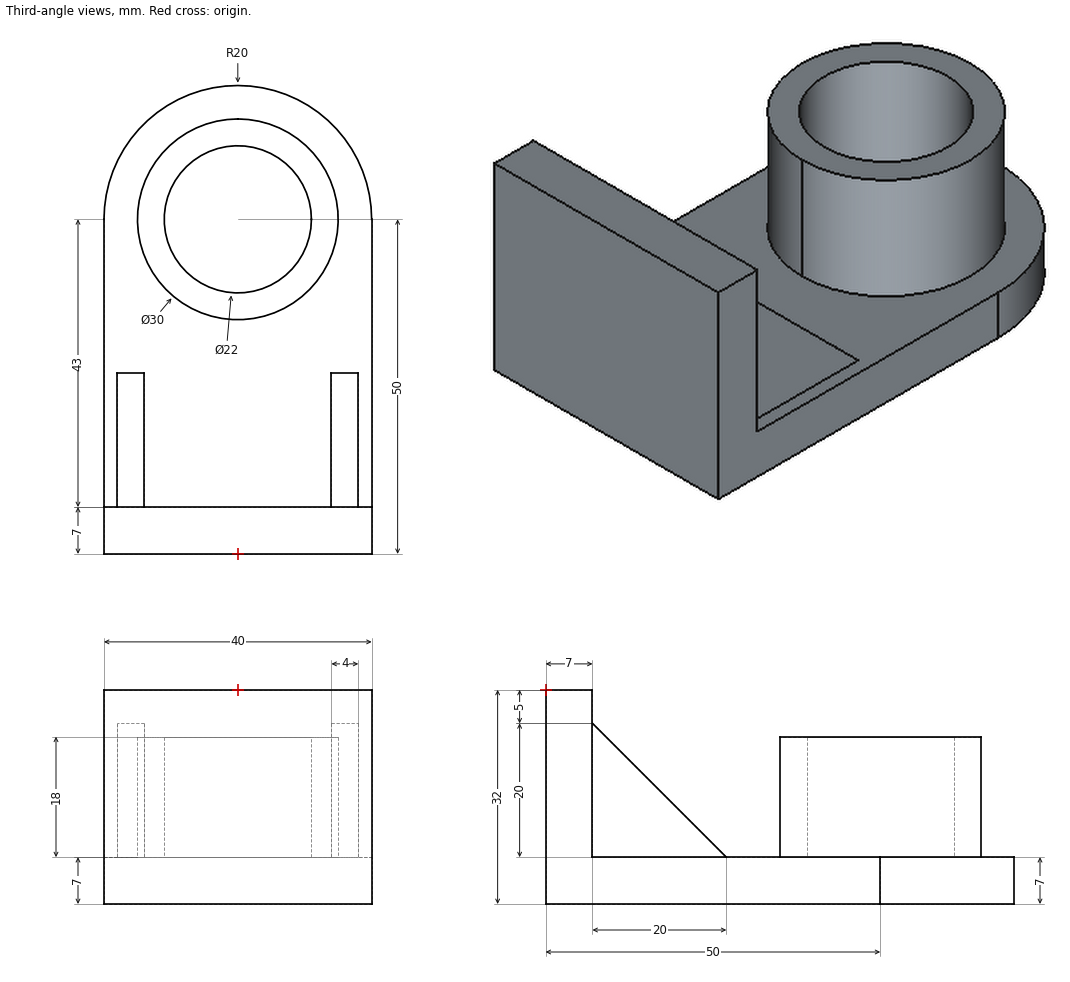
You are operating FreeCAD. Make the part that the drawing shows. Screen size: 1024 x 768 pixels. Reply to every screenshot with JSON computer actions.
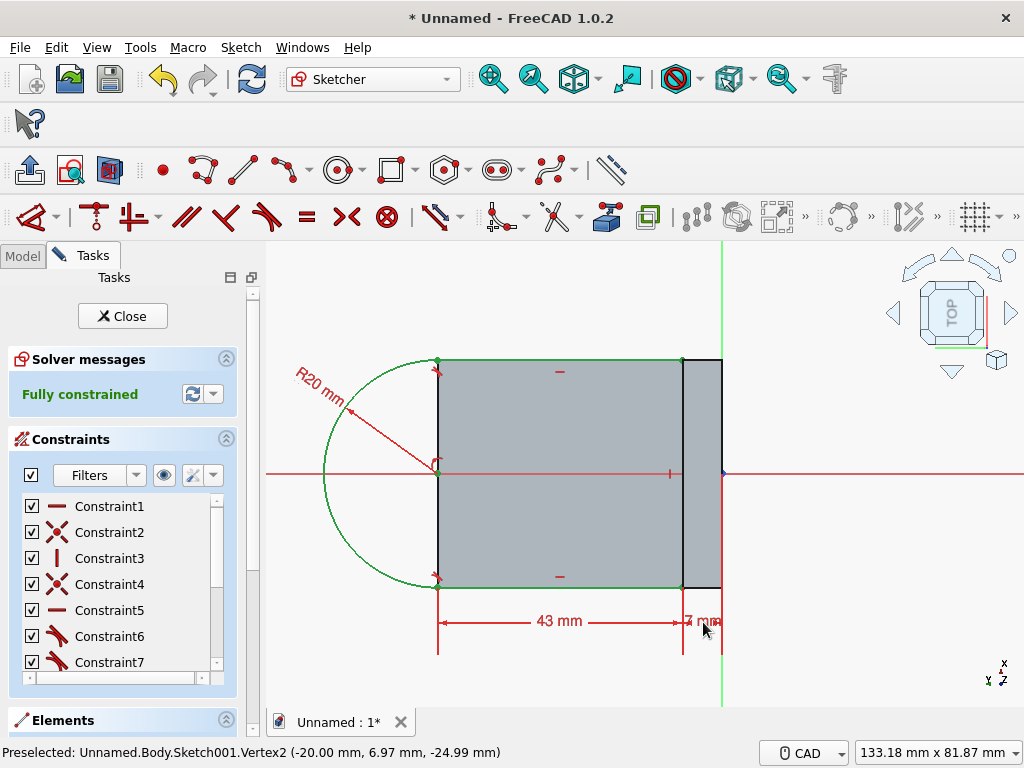
{"action": "left_click", "coordinate": [123, 316]}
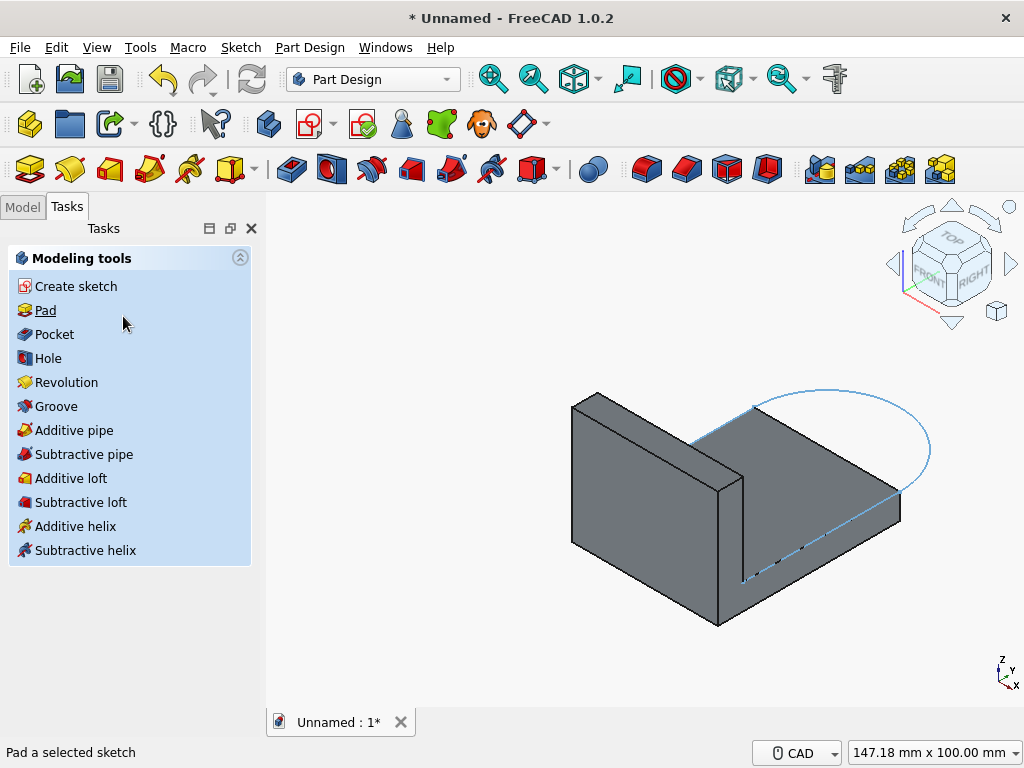
{"action": "left_click", "coordinate": [30, 170]}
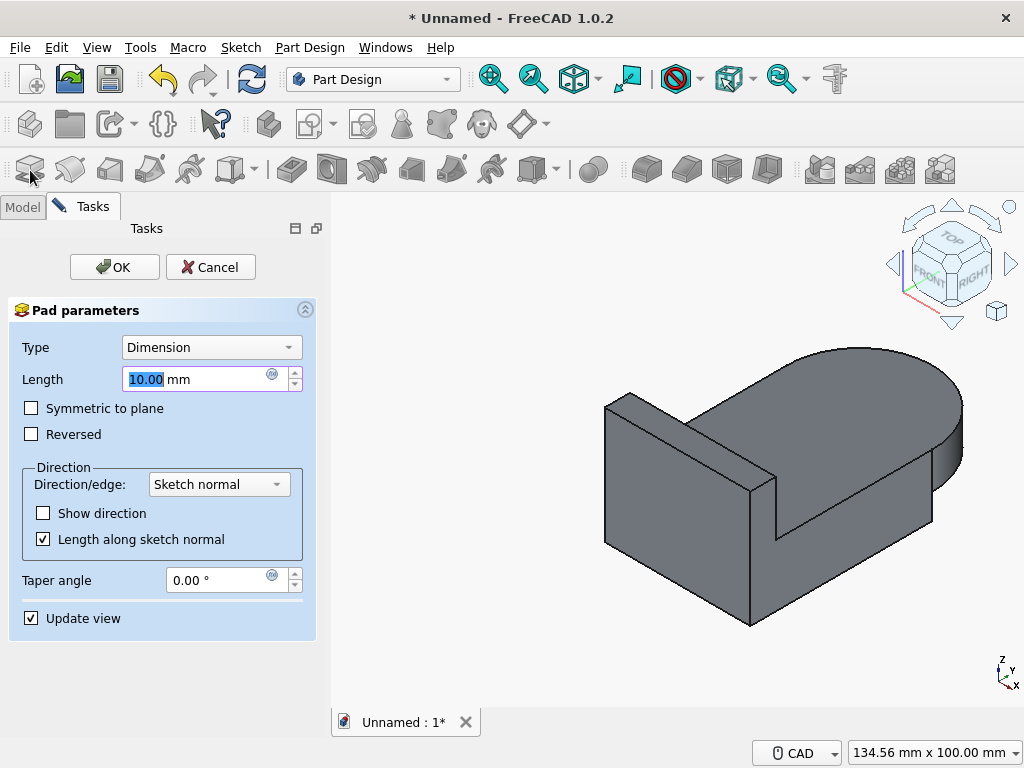
{"action": "type", "text": "7"}
{"action": "key", "text": "Tab"}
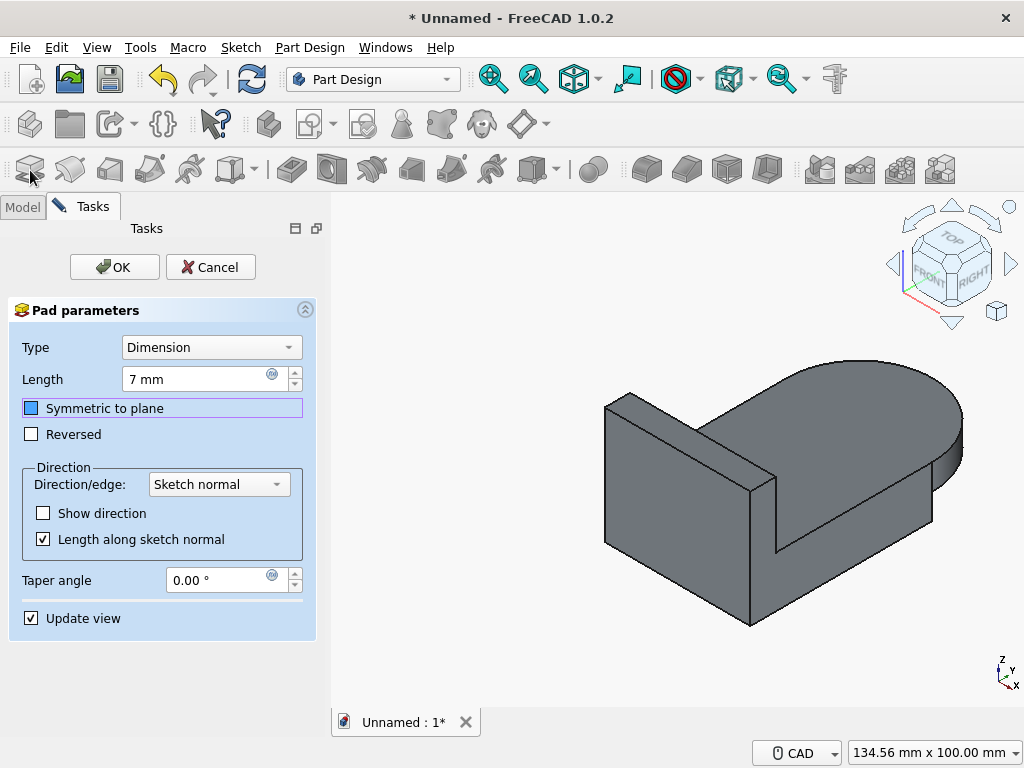
{"action": "left_click", "coordinate": [30, 434]}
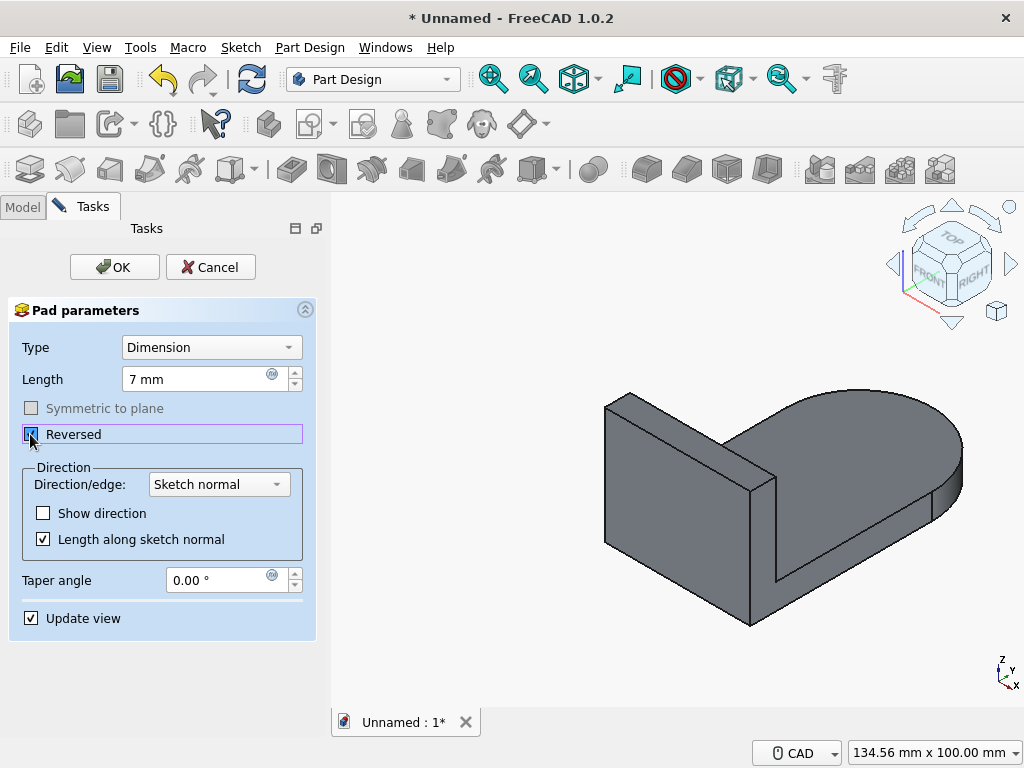
{"action": "left_click", "coordinate": [115, 267]}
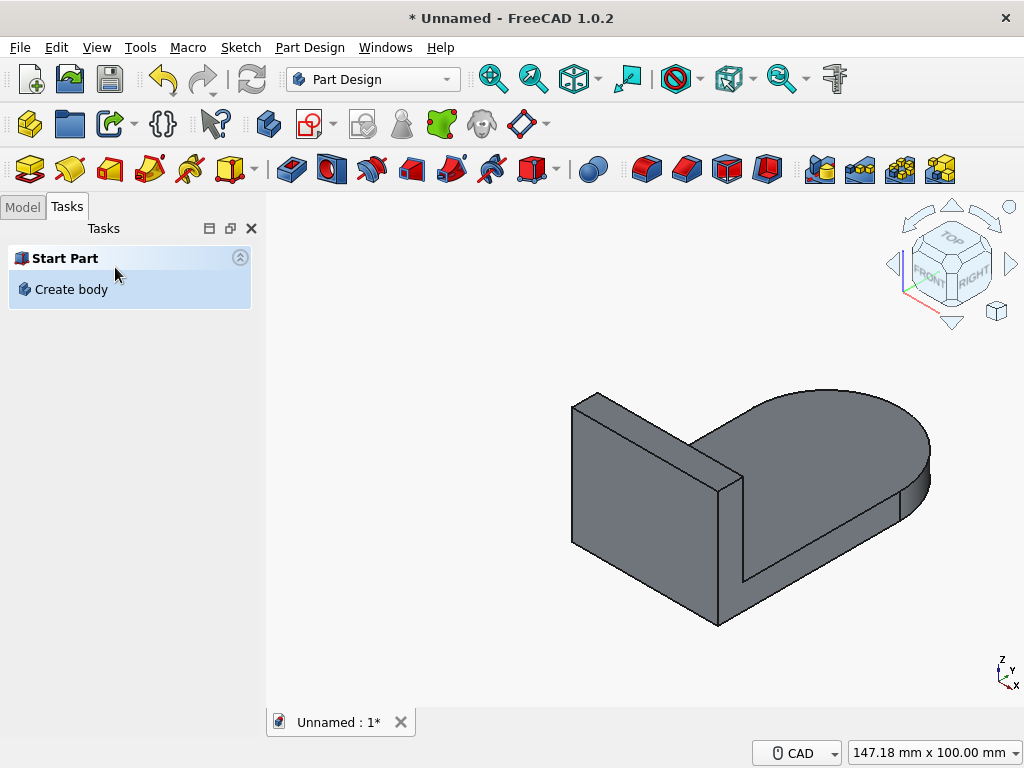
{"action": "left_click", "coordinate": [818, 454]}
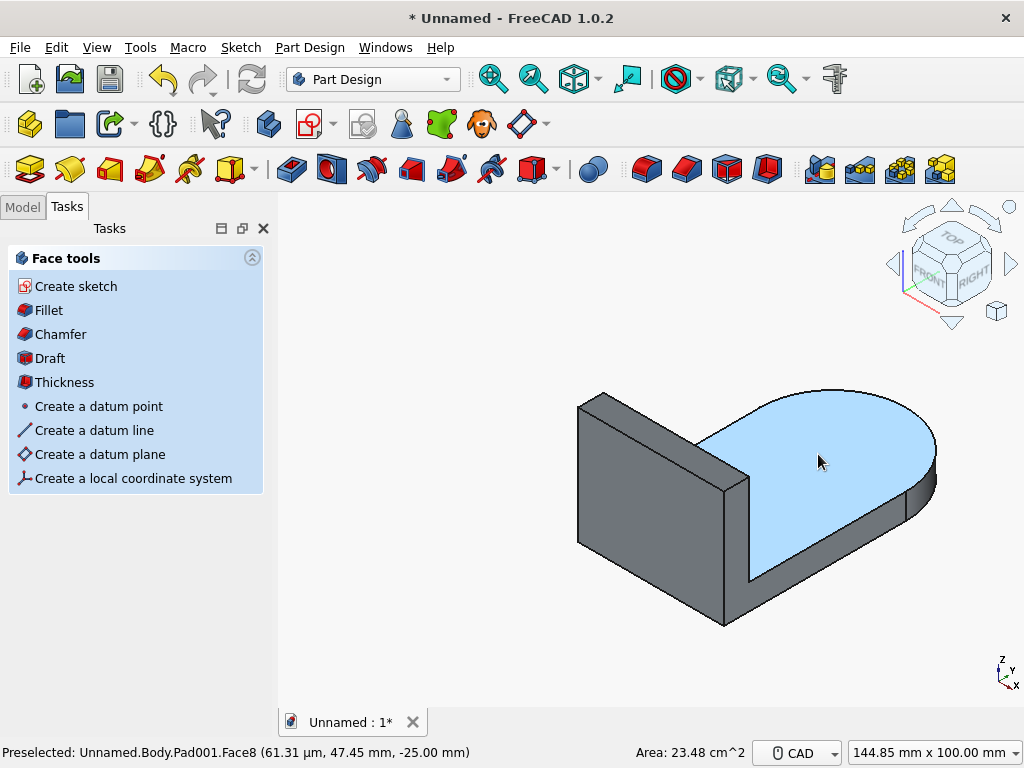
{"action": "left_click", "coordinate": [310, 124]}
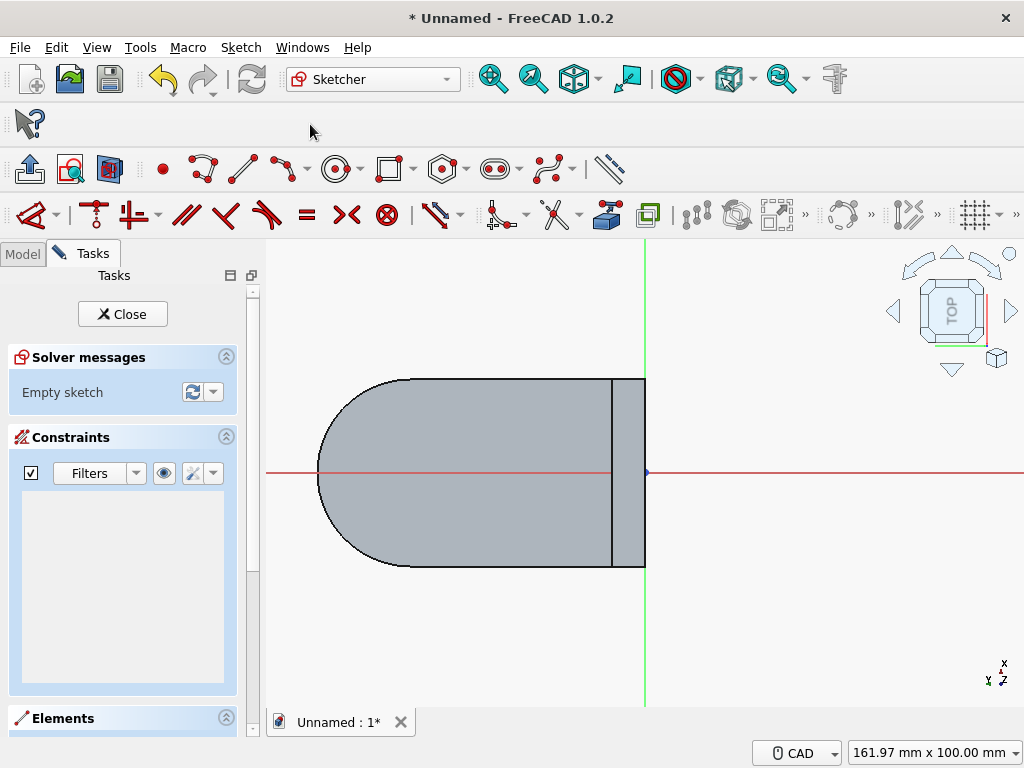
{"action": "key", "text": "g c"}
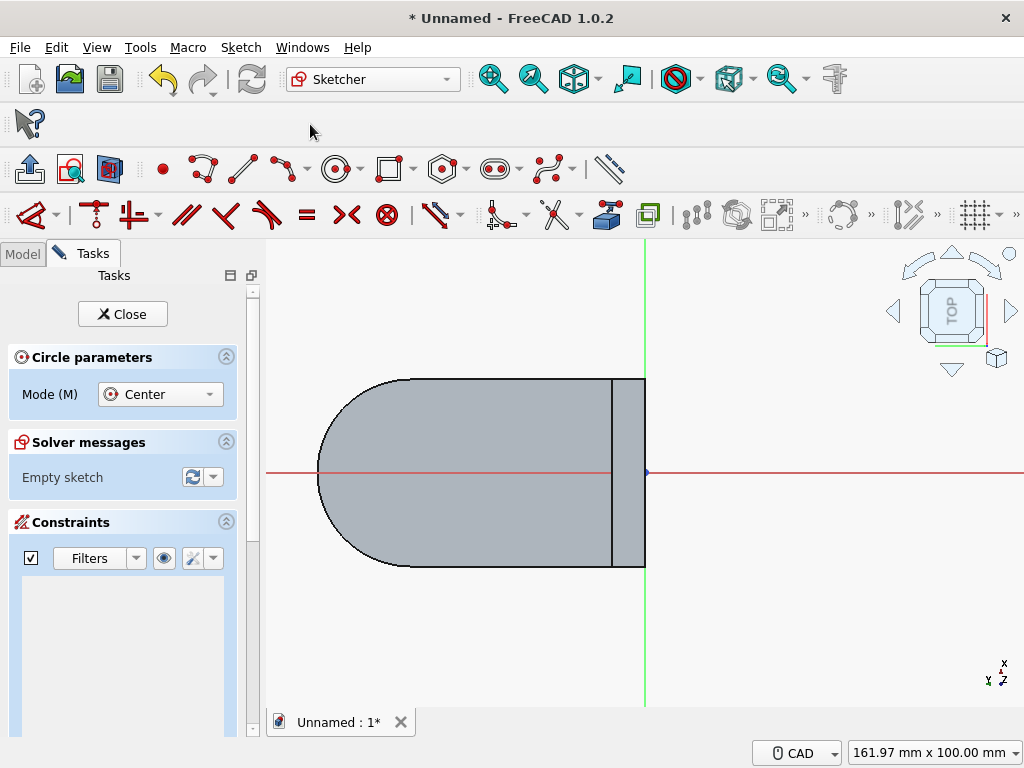
{"action": "left_click", "coordinate": [411, 473]}
{"action": "mouse_move", "coordinate": [461, 423]}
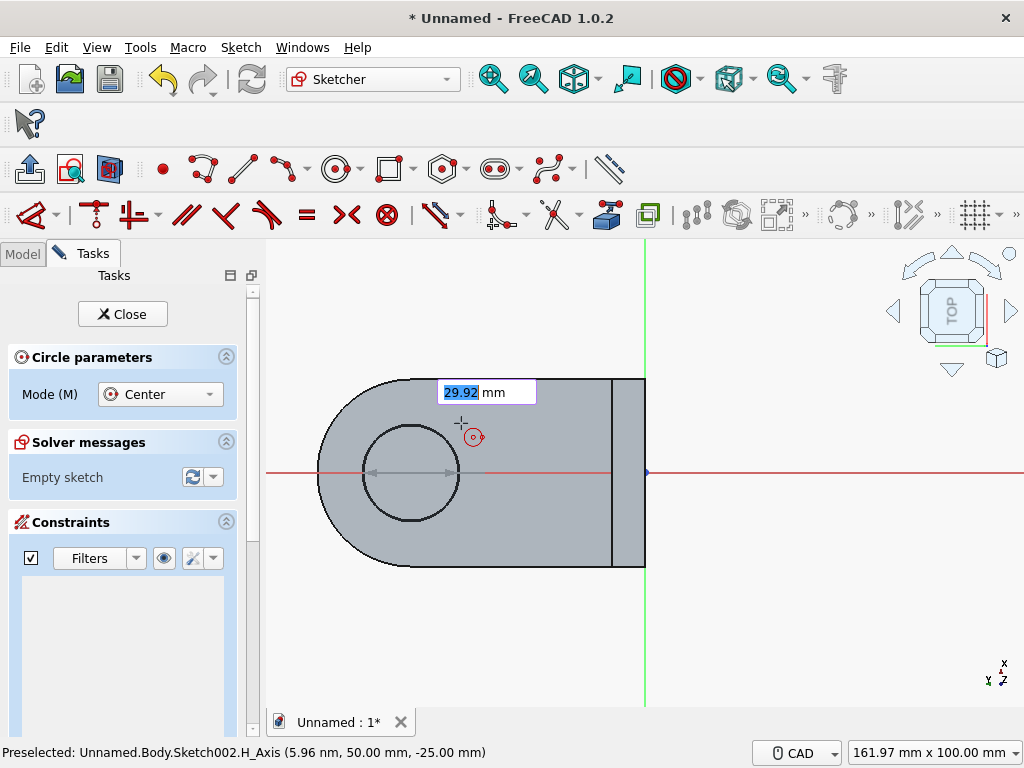
{"action": "type", "text": "30"}
{"action": "key", "text": "Return"}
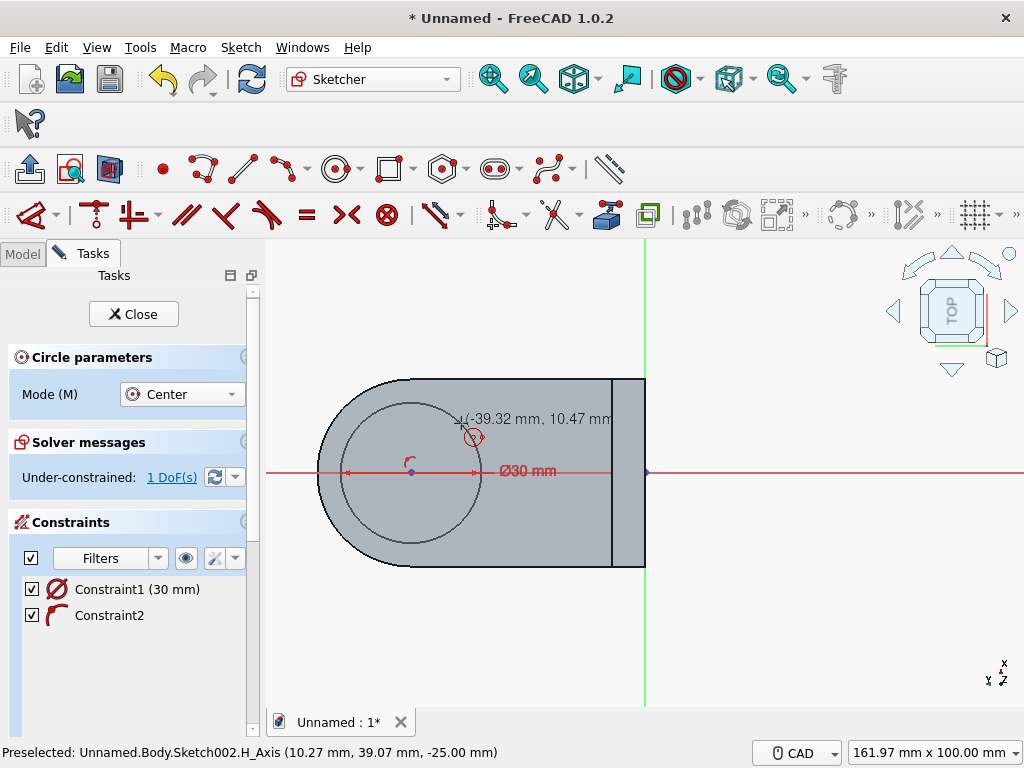
{"action": "left_click", "coordinate": [411, 473]}
{"action": "mouse_move", "coordinate": [447, 437]}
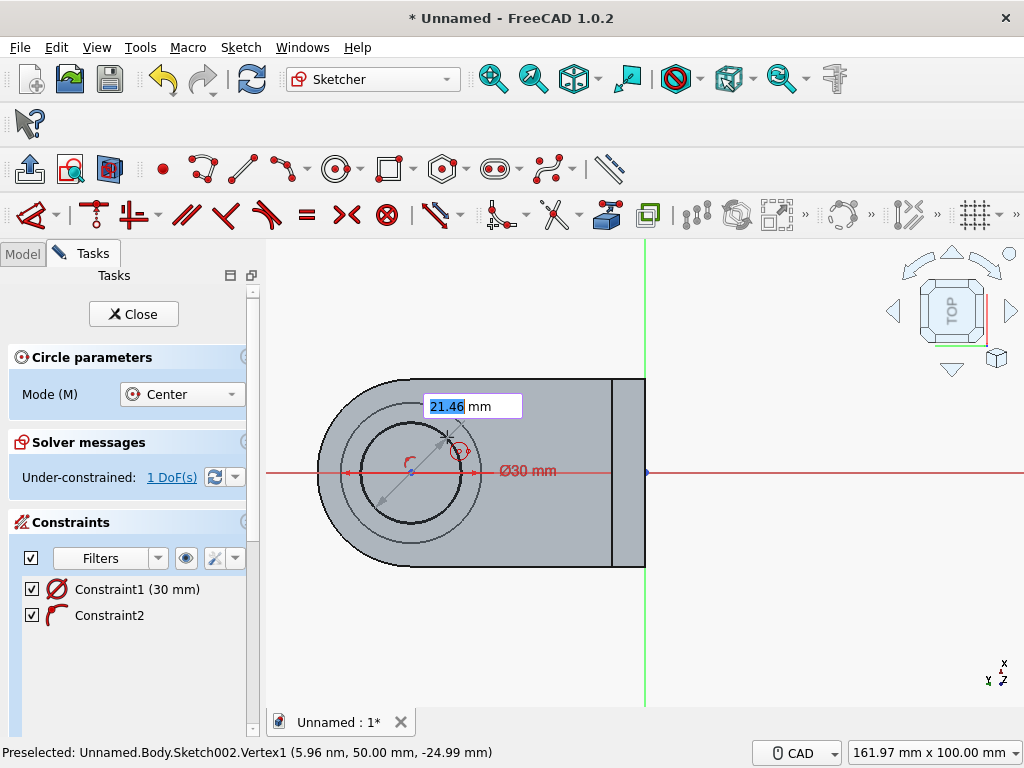
{"action": "type", "text": "22"}
{"action": "key", "text": "Return"}
{"action": "key", "text": "Escape"}